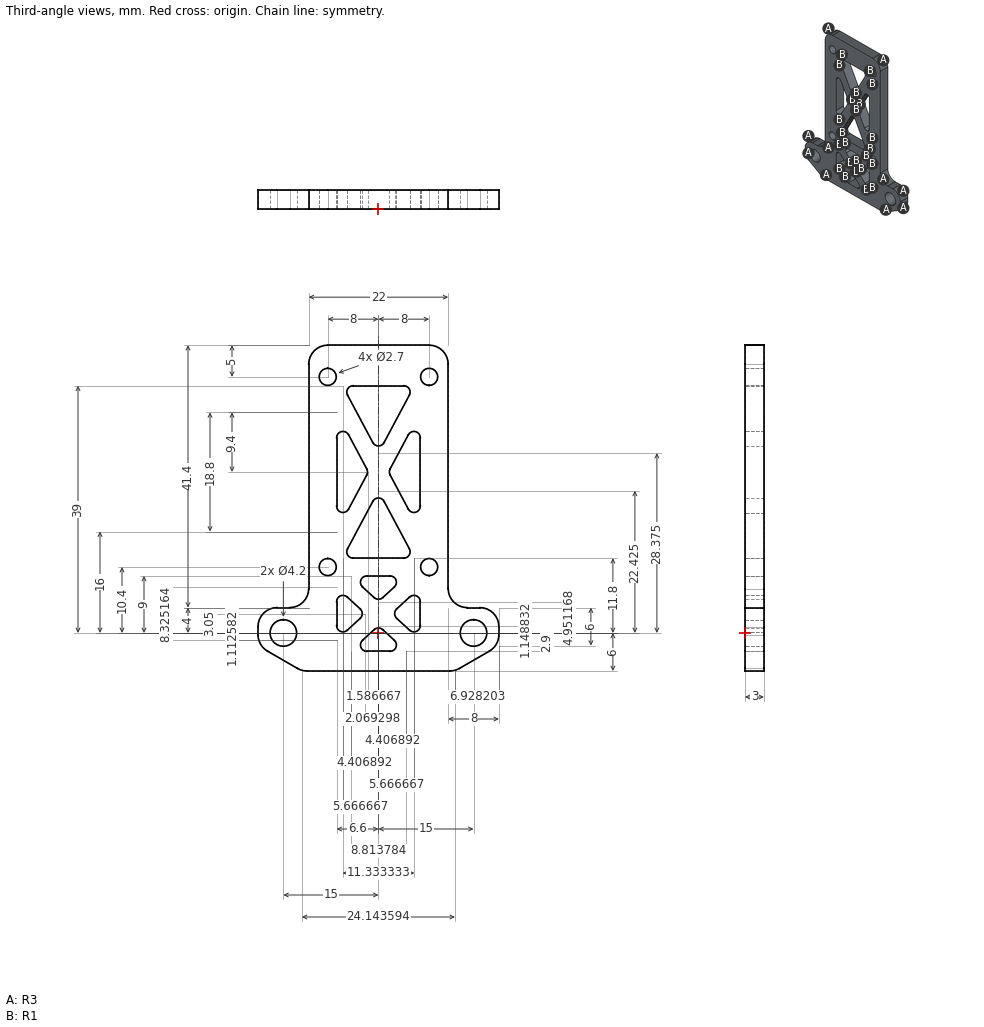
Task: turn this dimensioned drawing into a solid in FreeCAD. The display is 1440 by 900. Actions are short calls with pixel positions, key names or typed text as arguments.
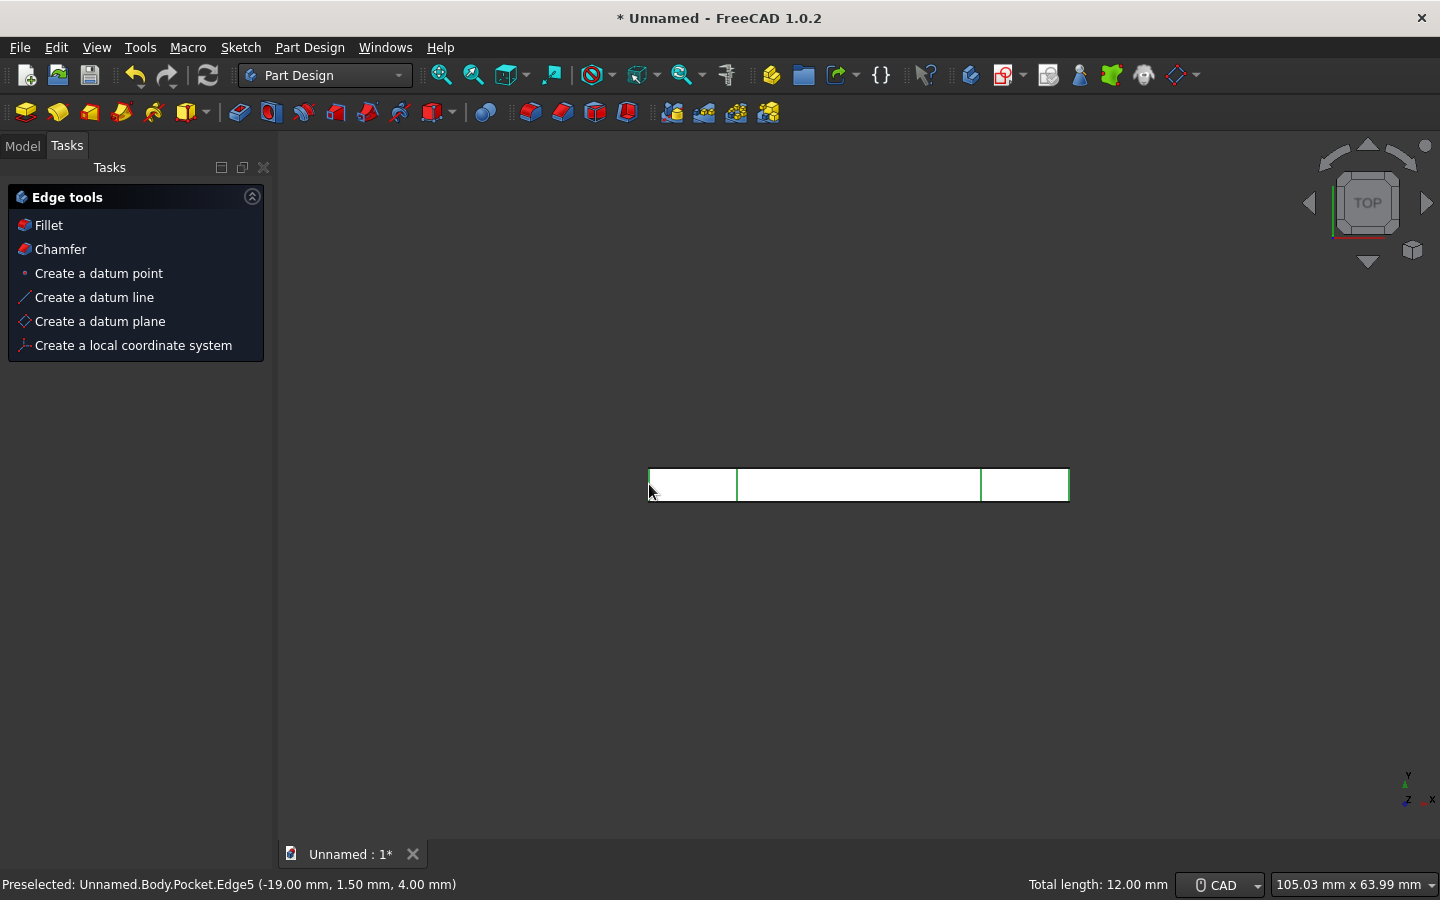
key(1)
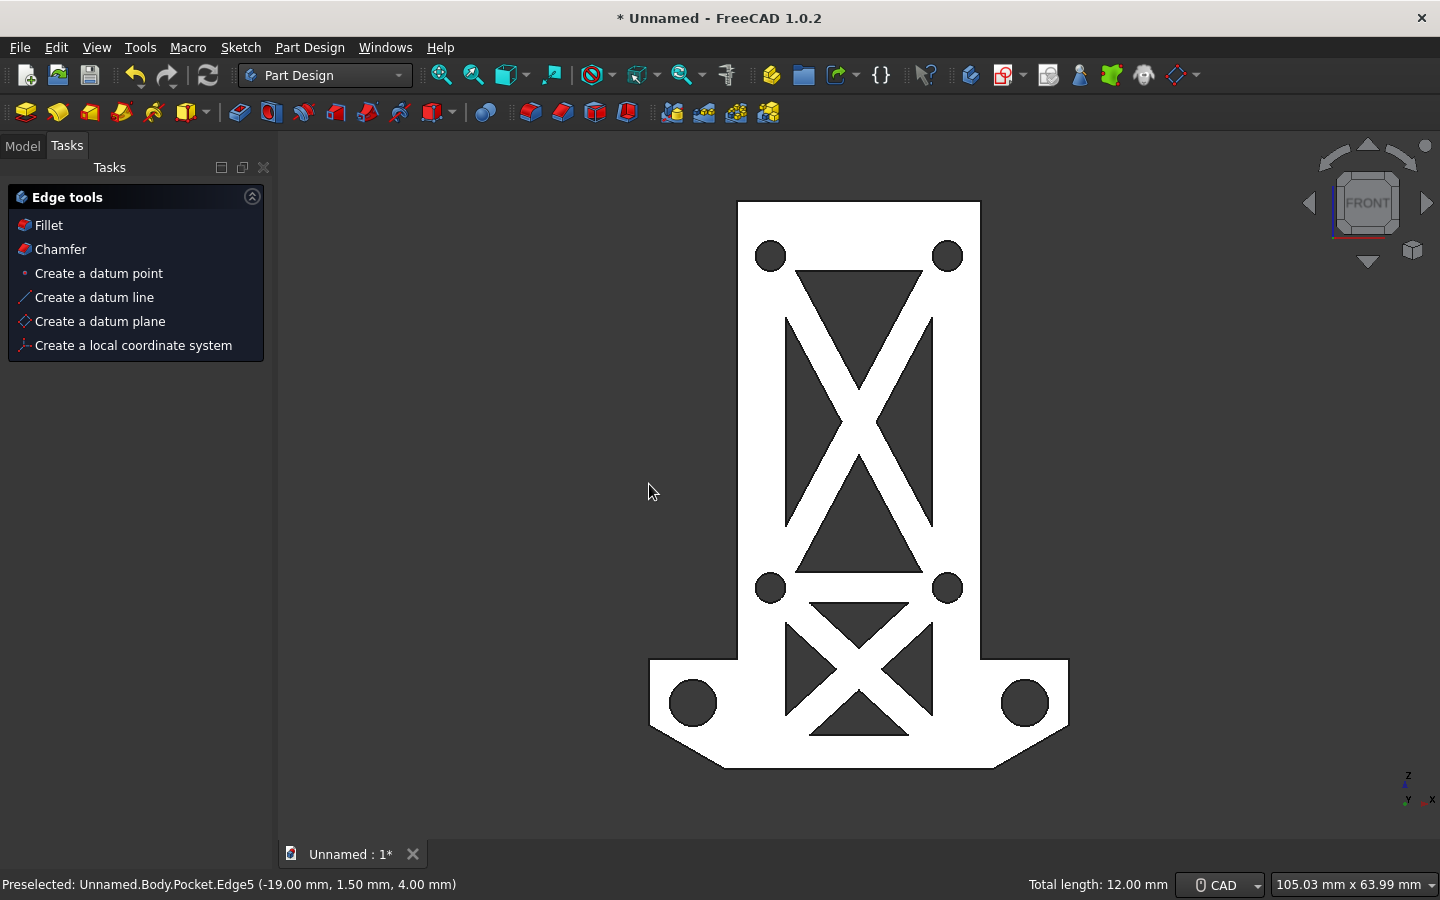
key(3)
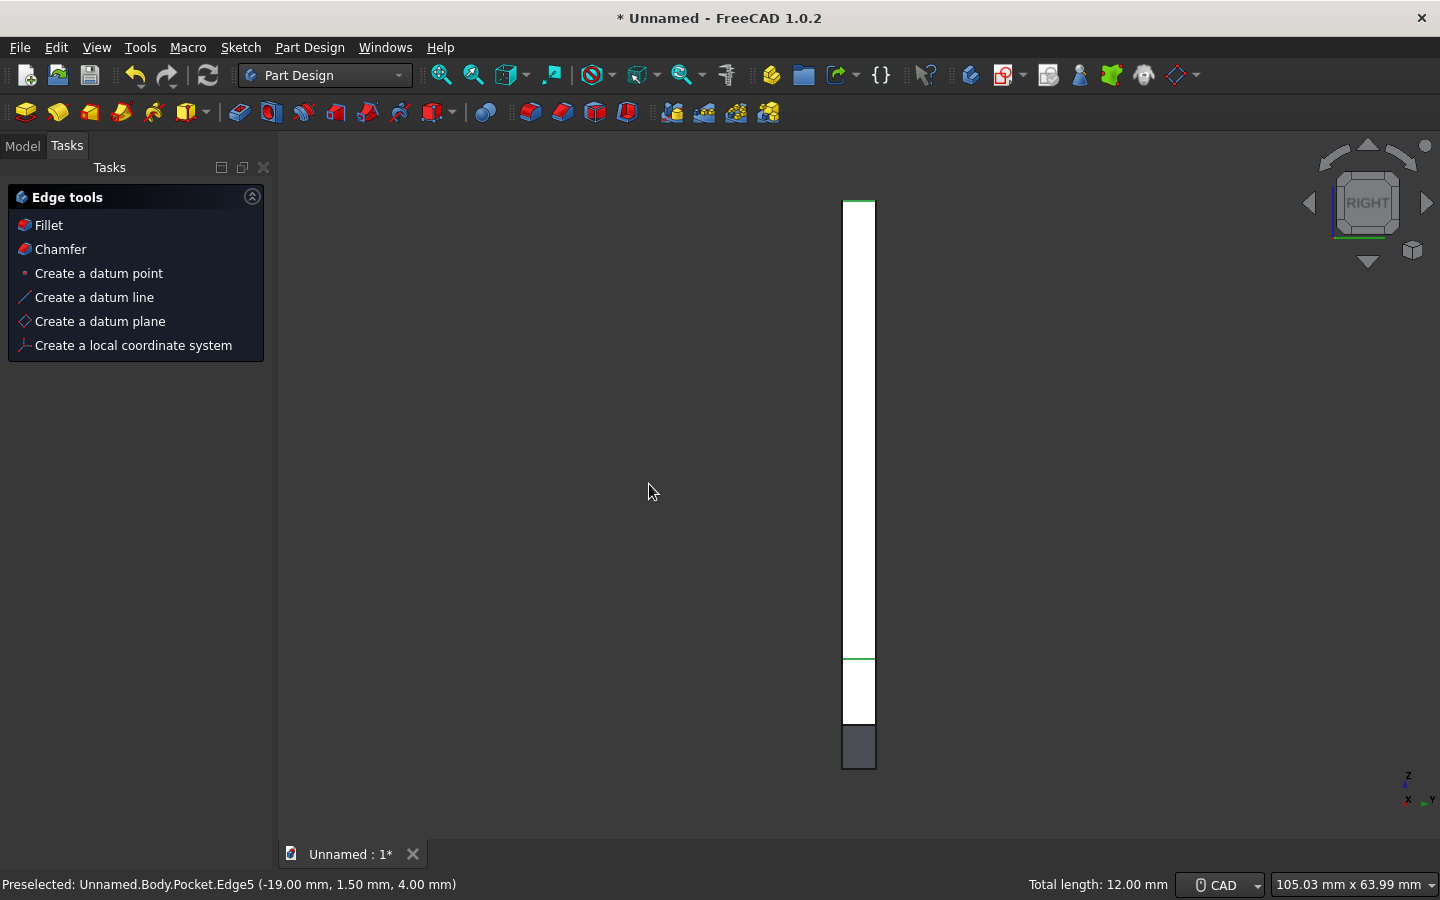
click(859, 724, ctrl)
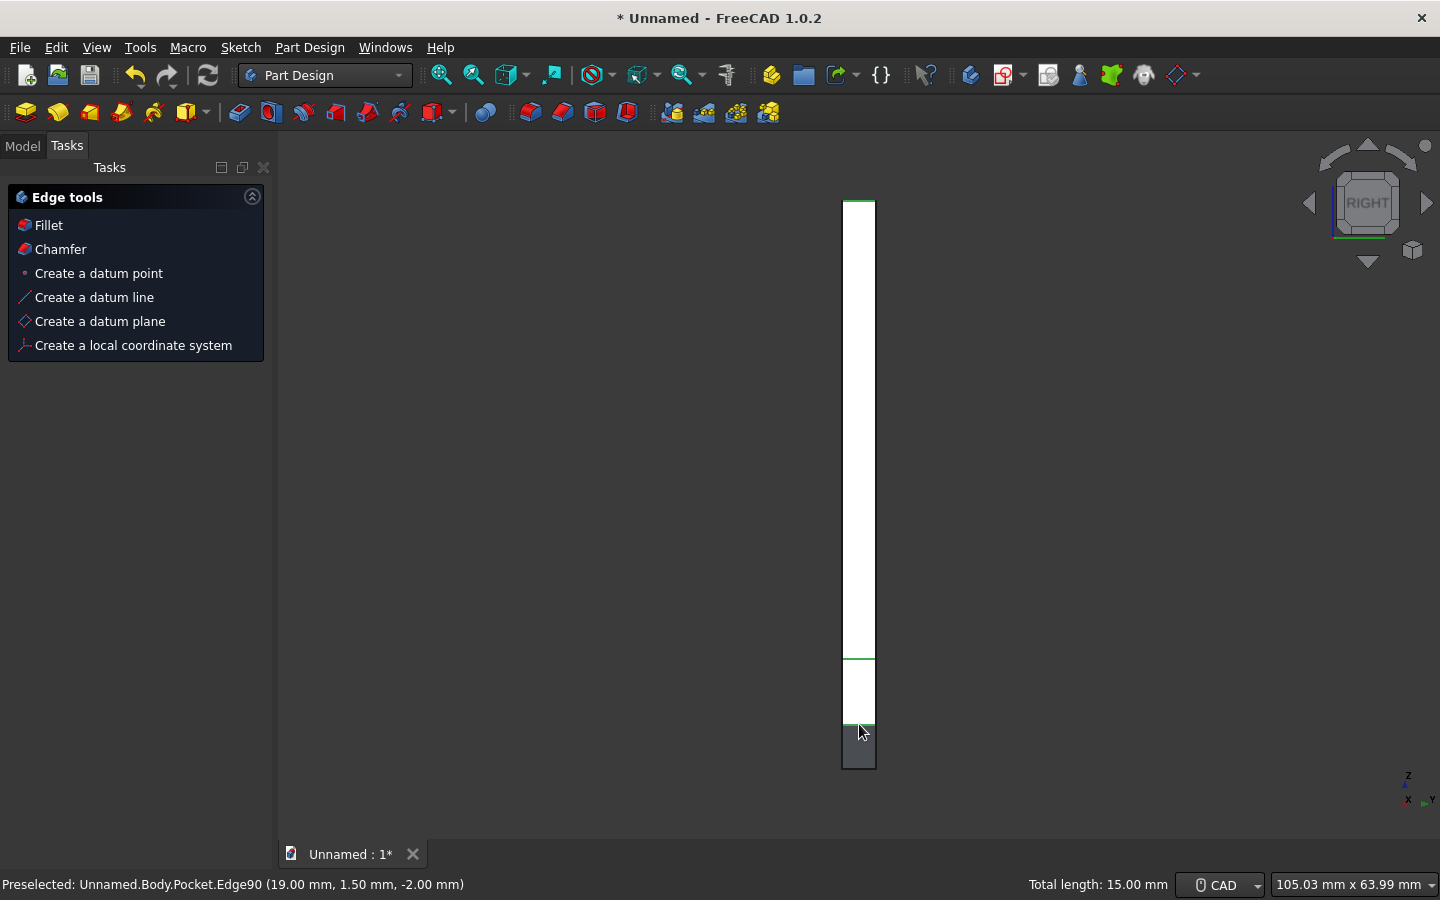
key(5)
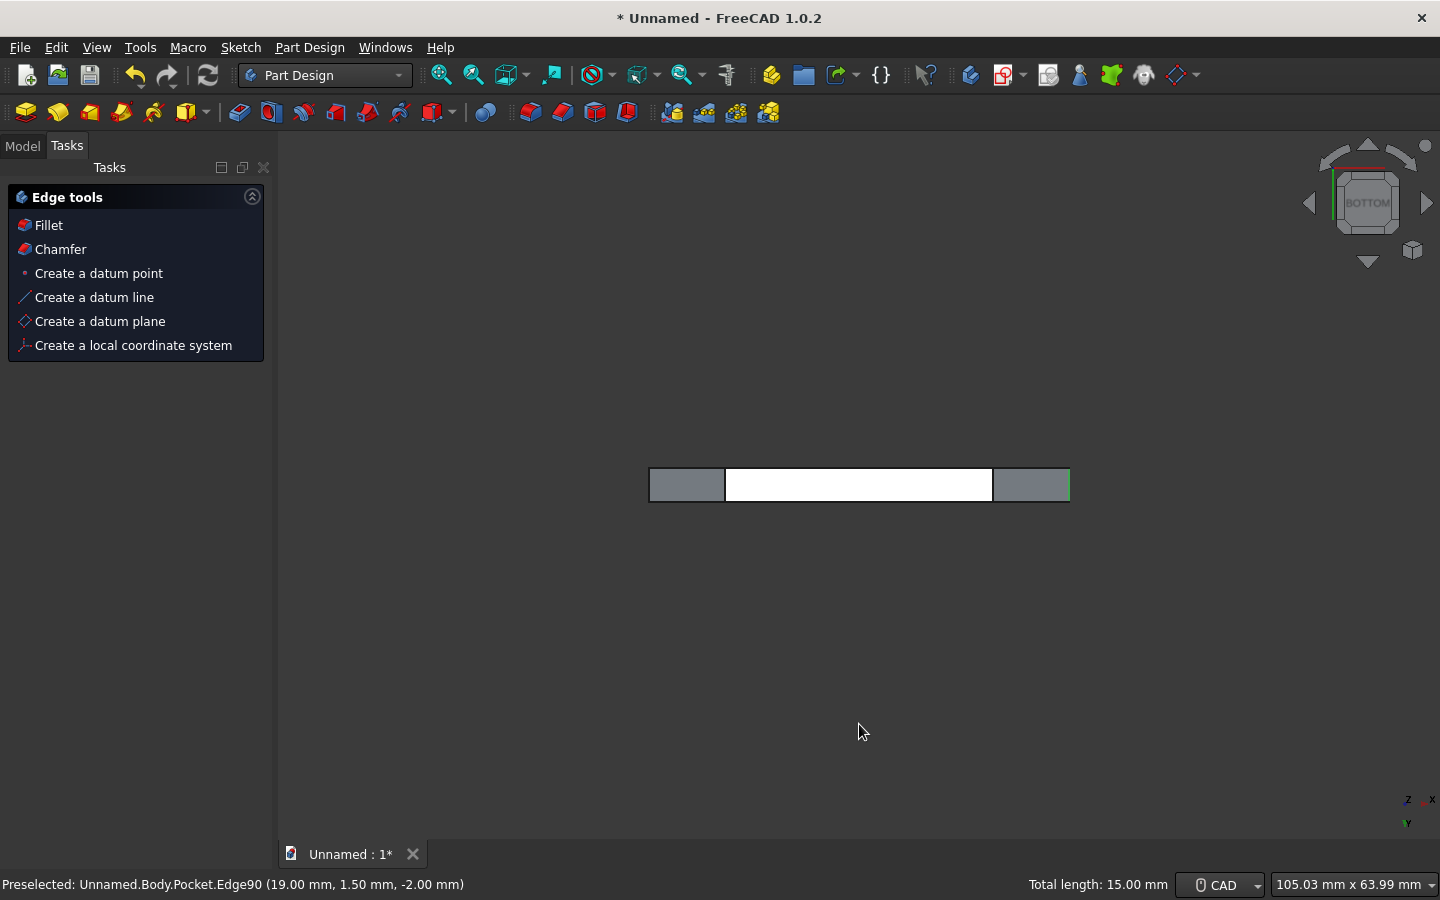
click(442, 76)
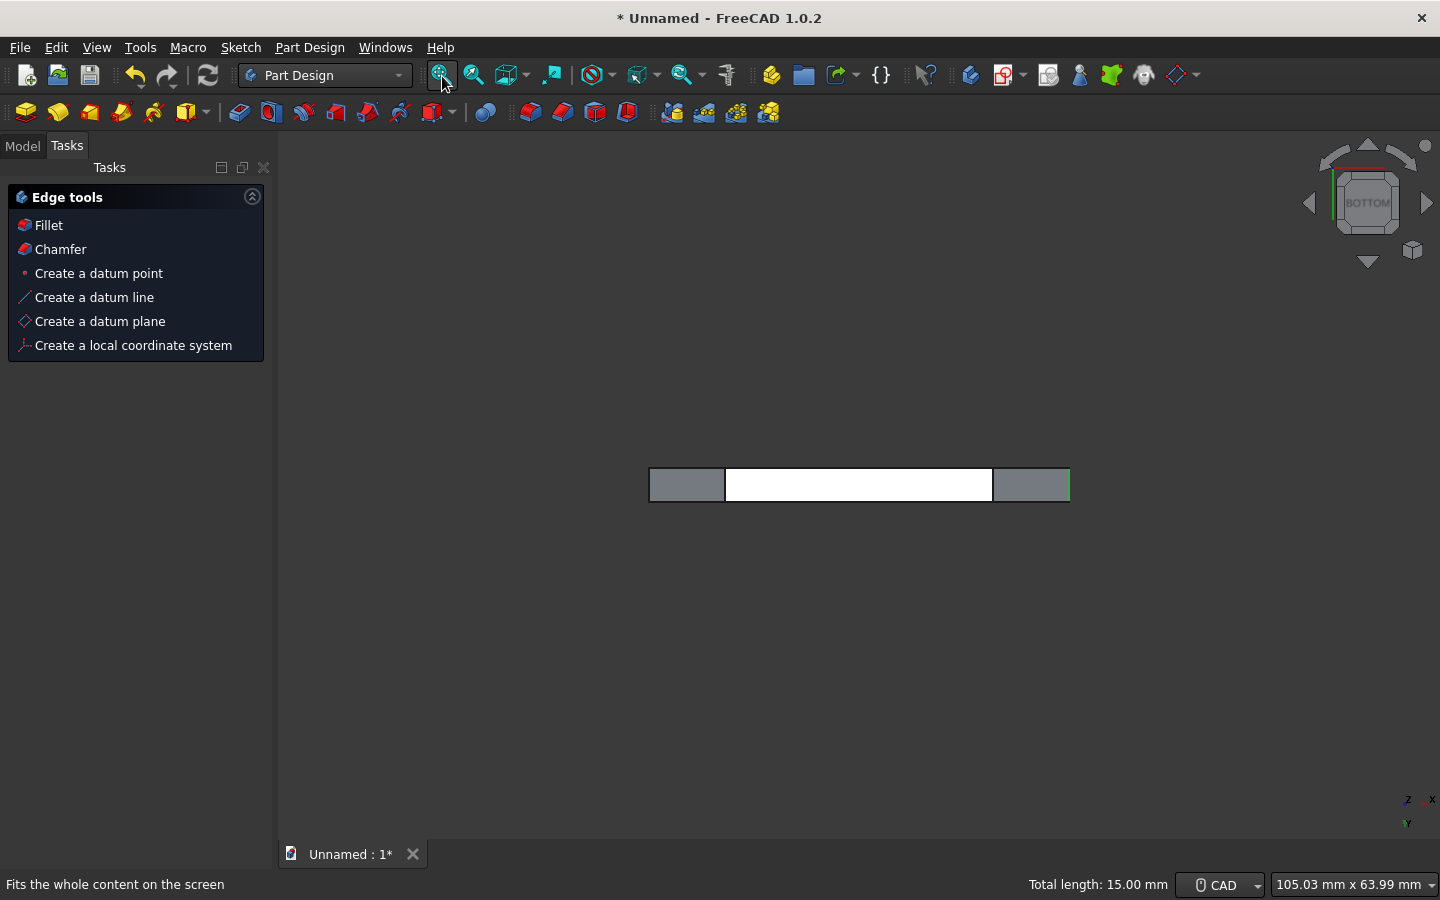
click(725, 484, ctrl)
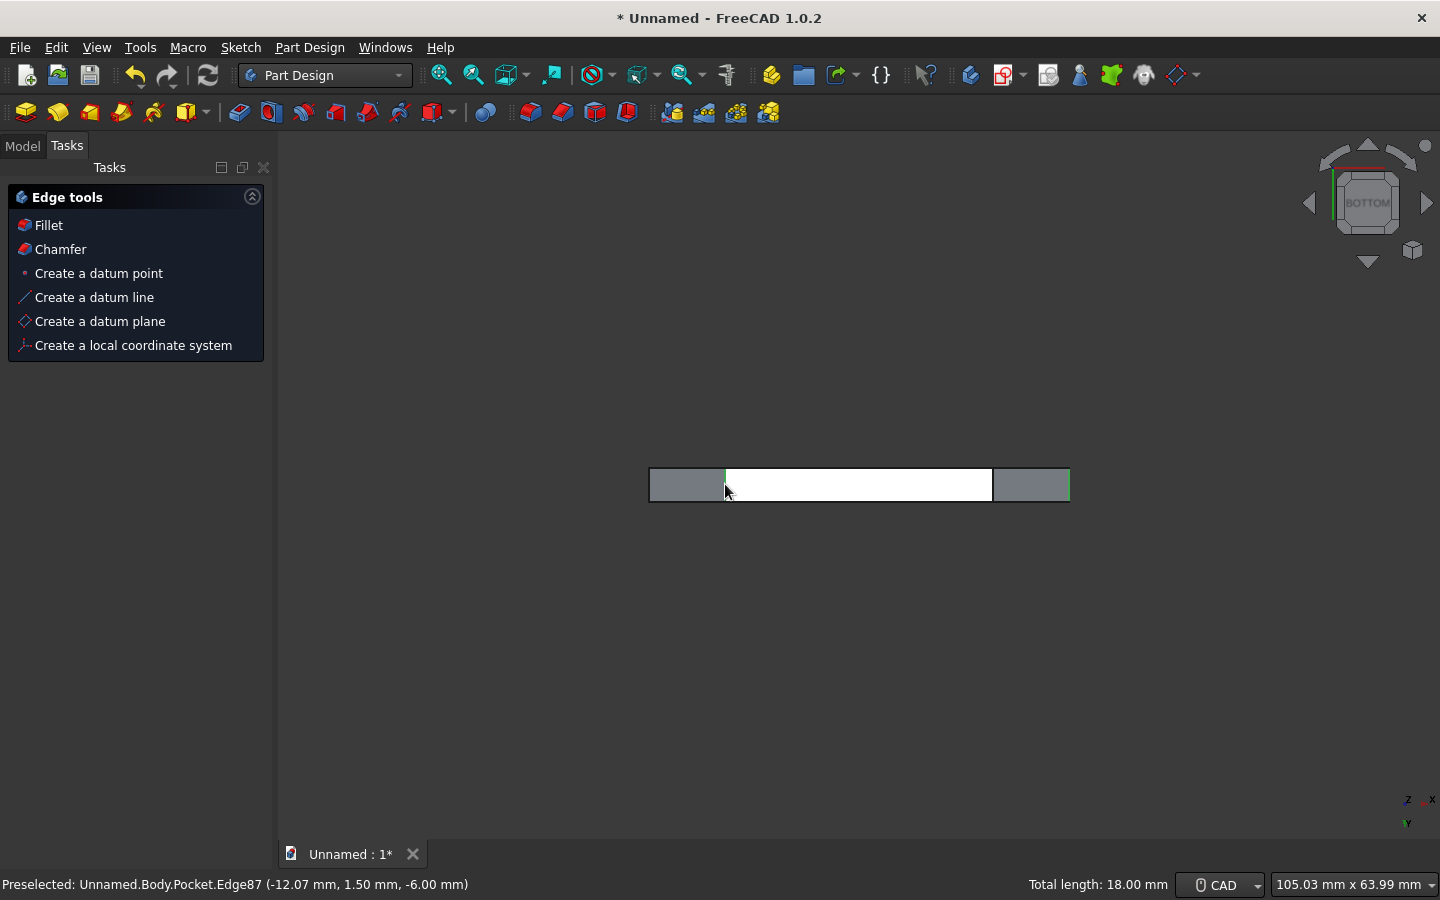
click(993, 484, ctrl)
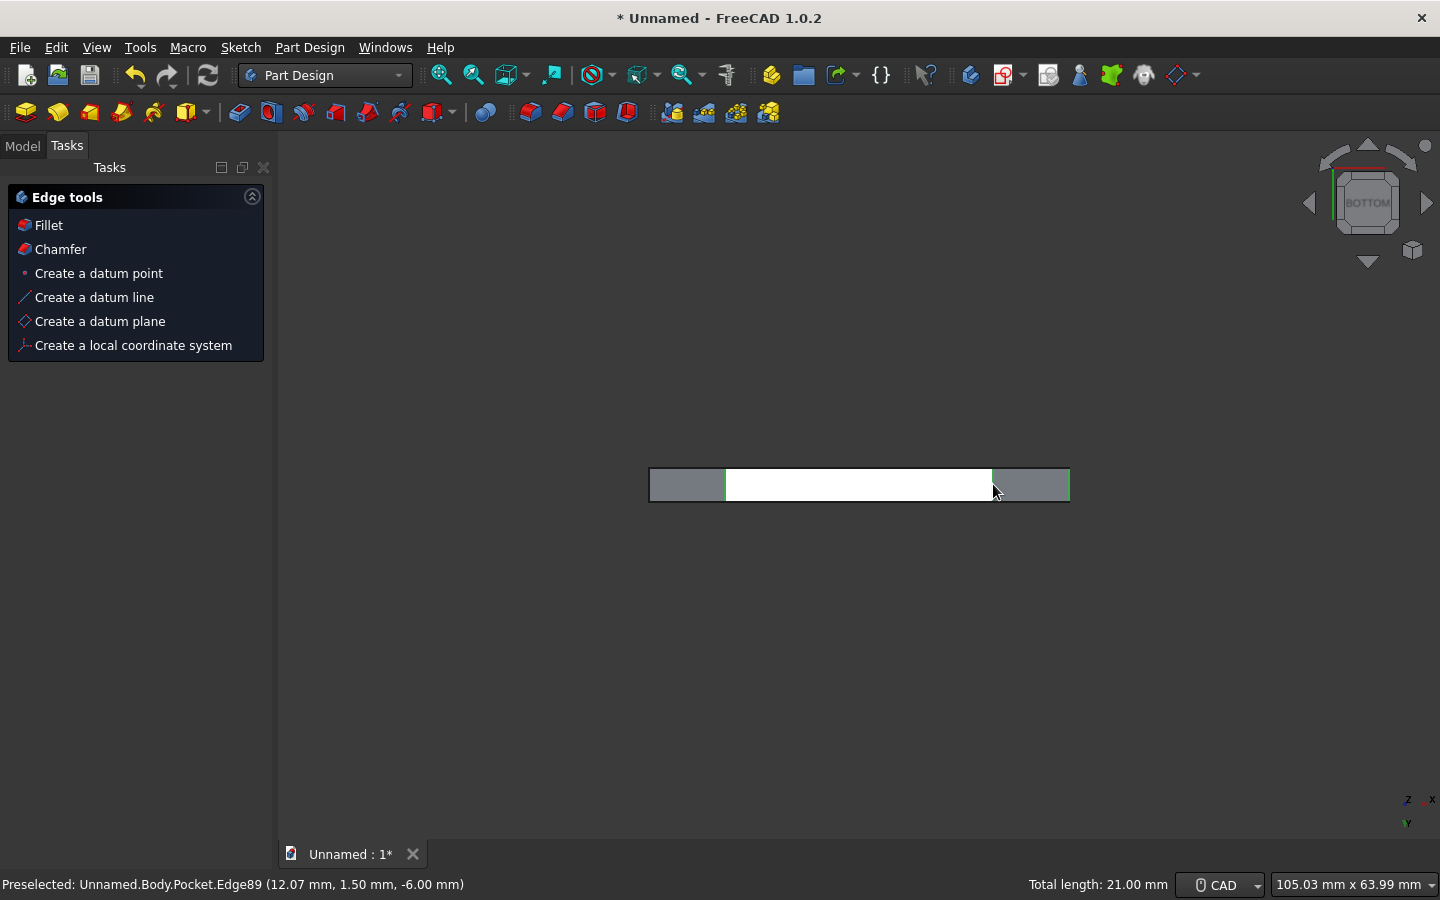
key(4)